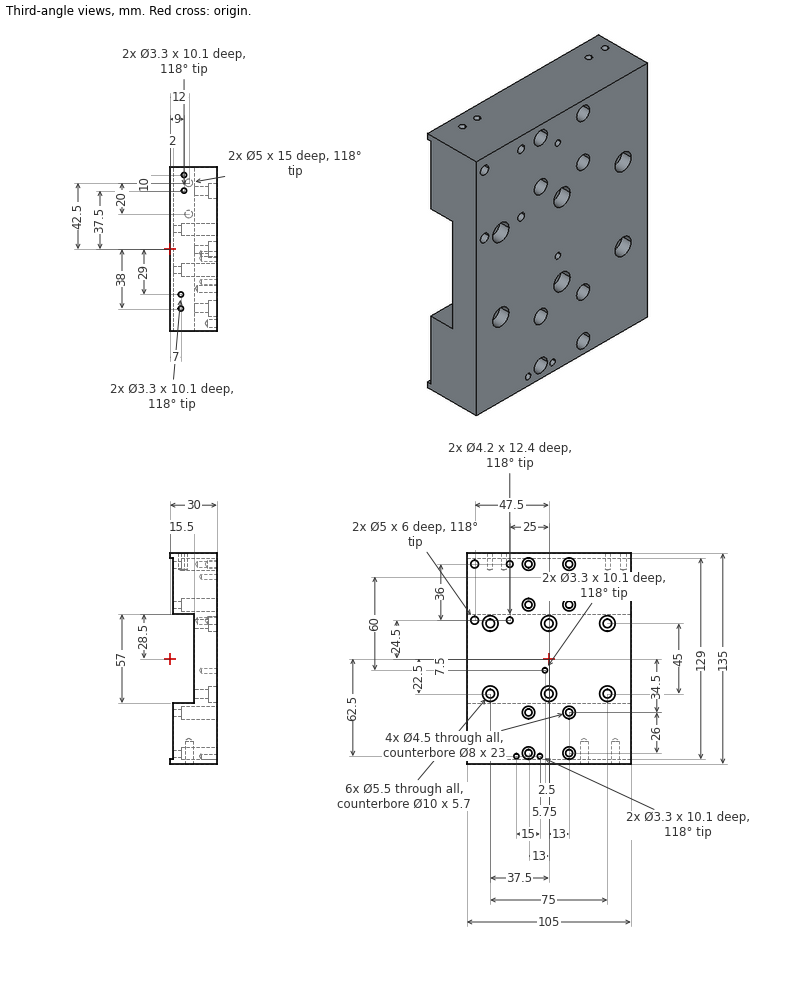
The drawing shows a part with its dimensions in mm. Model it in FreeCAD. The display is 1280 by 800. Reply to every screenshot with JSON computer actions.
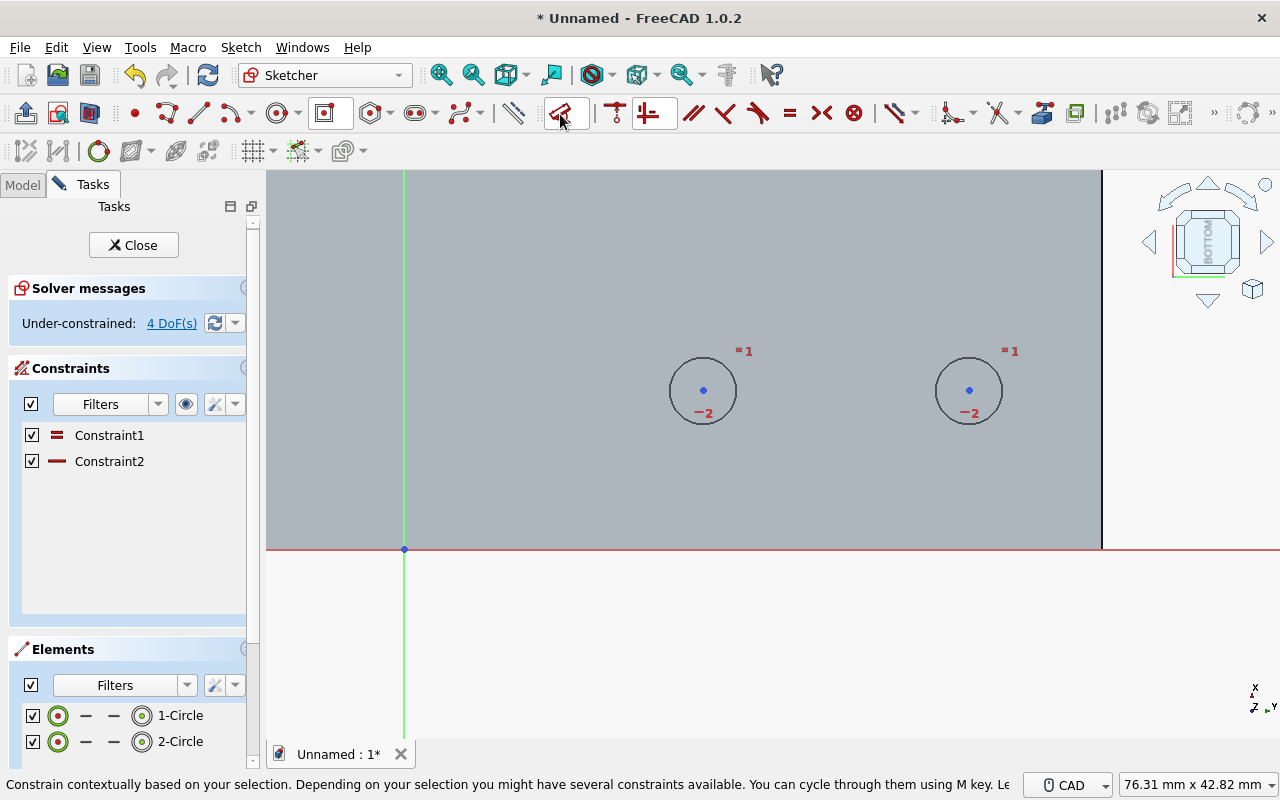
{"action": "left_click", "coordinate": [992, 367]}
{"action": "left_click", "coordinate": [1014, 344]}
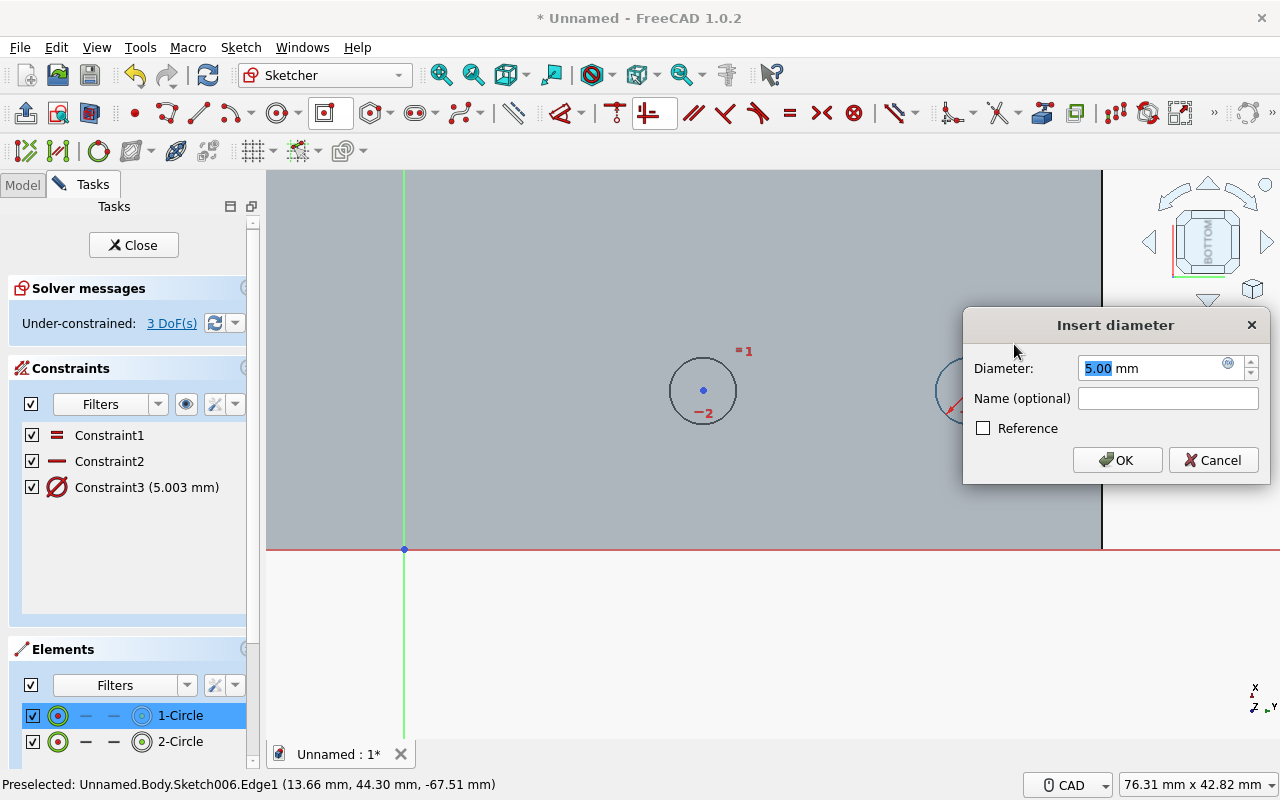
{"action": "type", "text": "5"}
{"action": "key", "text": "Return"}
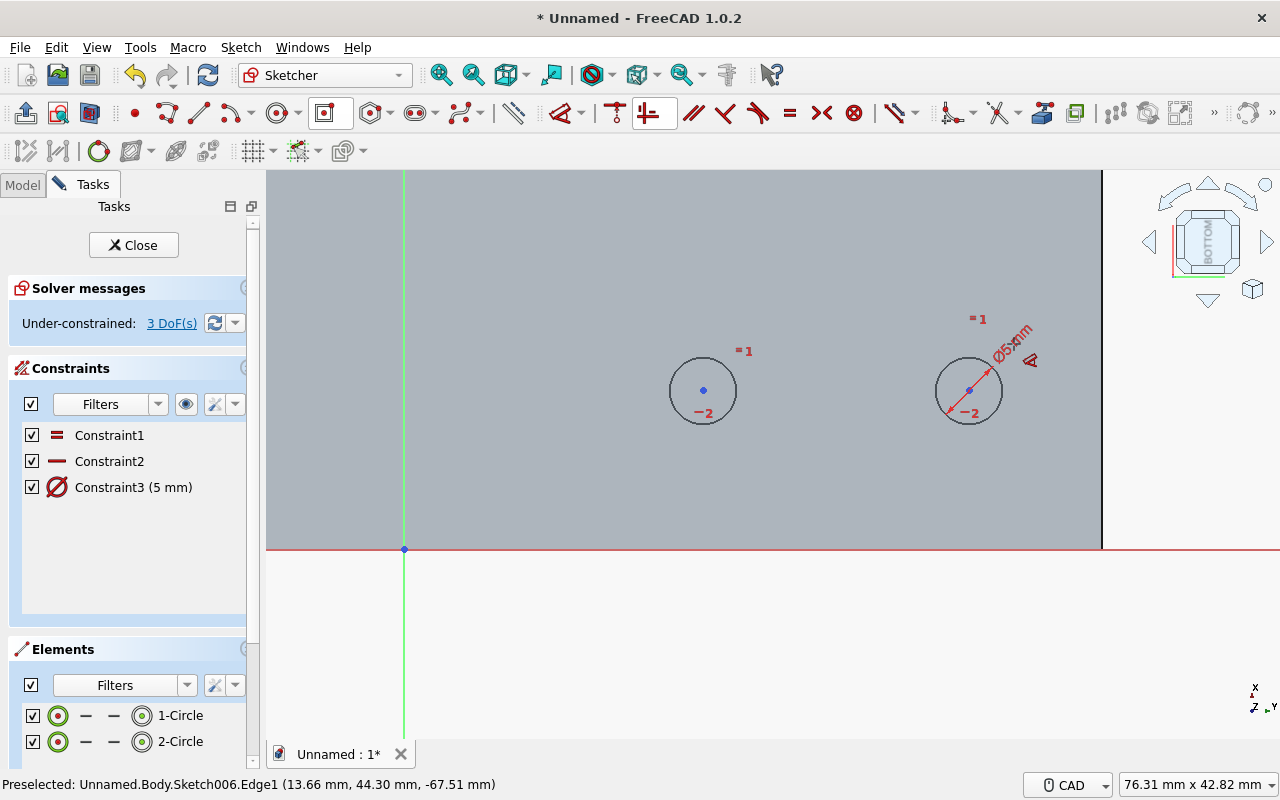
{"action": "left_click", "coordinate": [969, 391]}
{"action": "left_click", "coordinate": [370, 470]}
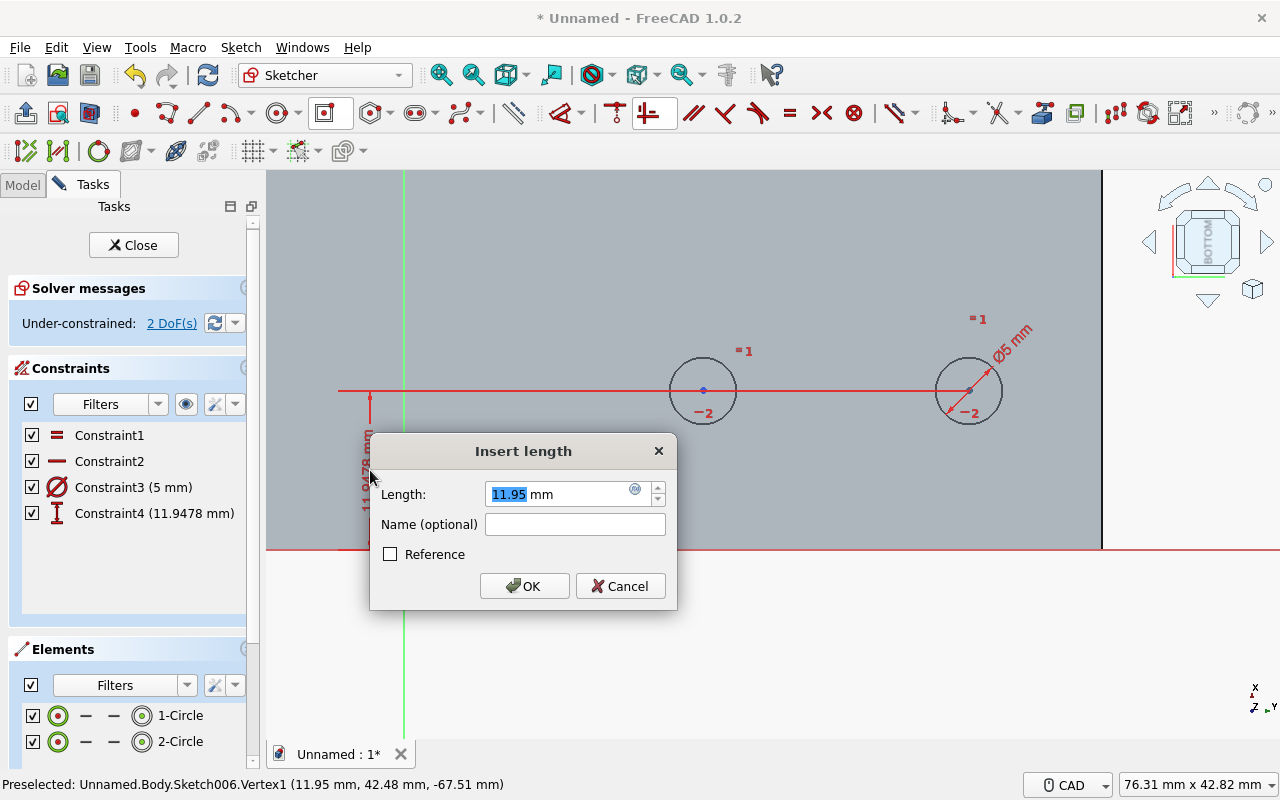
{"action": "type", "text": "12"}
{"action": "key", "text": "Return"}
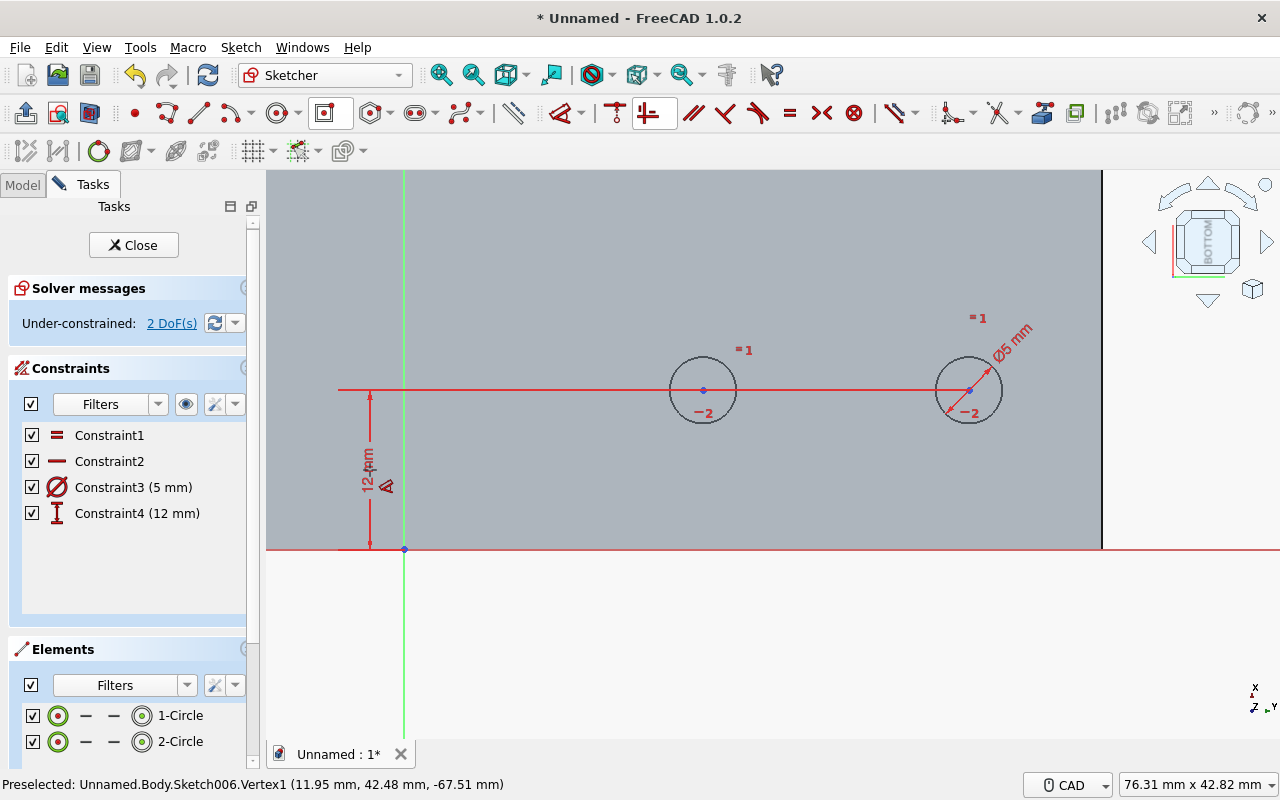
{"action": "left_click", "coordinate": [969, 390]}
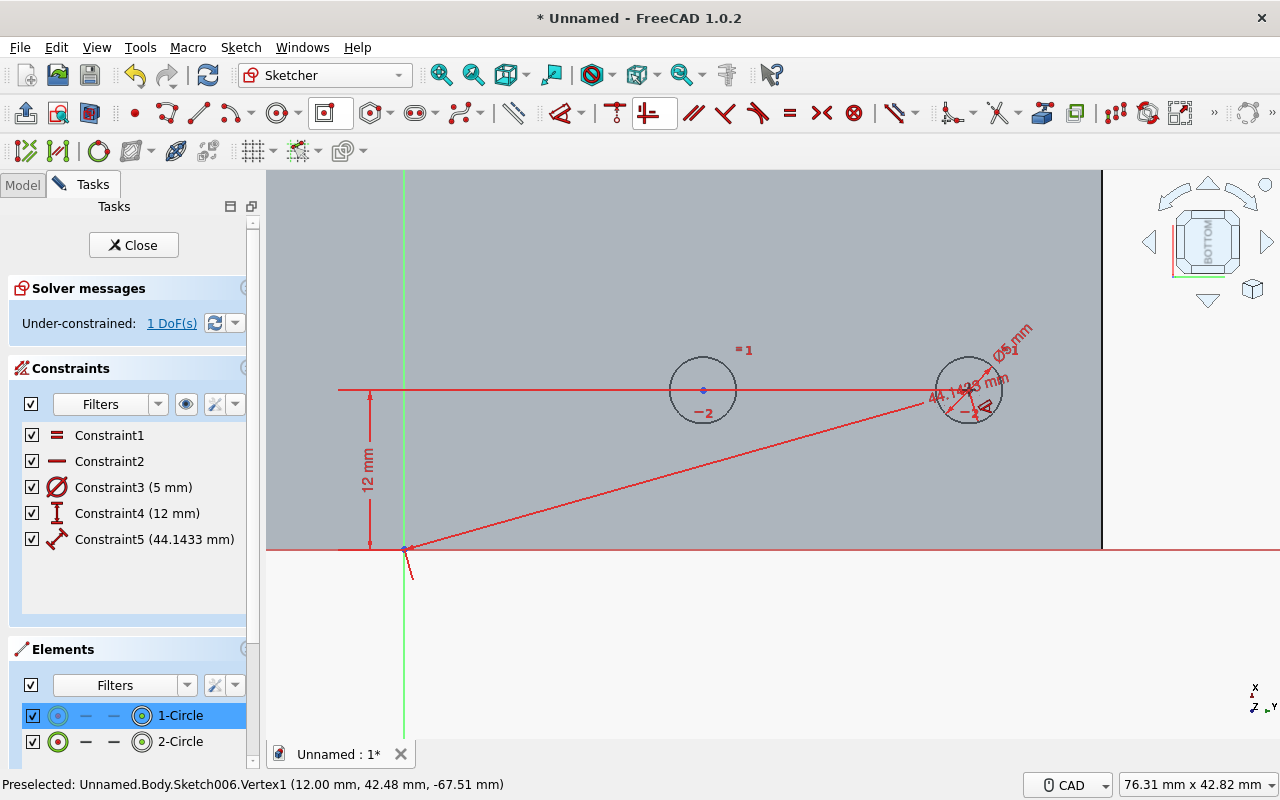
{"action": "left_click", "coordinate": [703, 390]}
{"action": "left_click", "coordinate": [836, 356]}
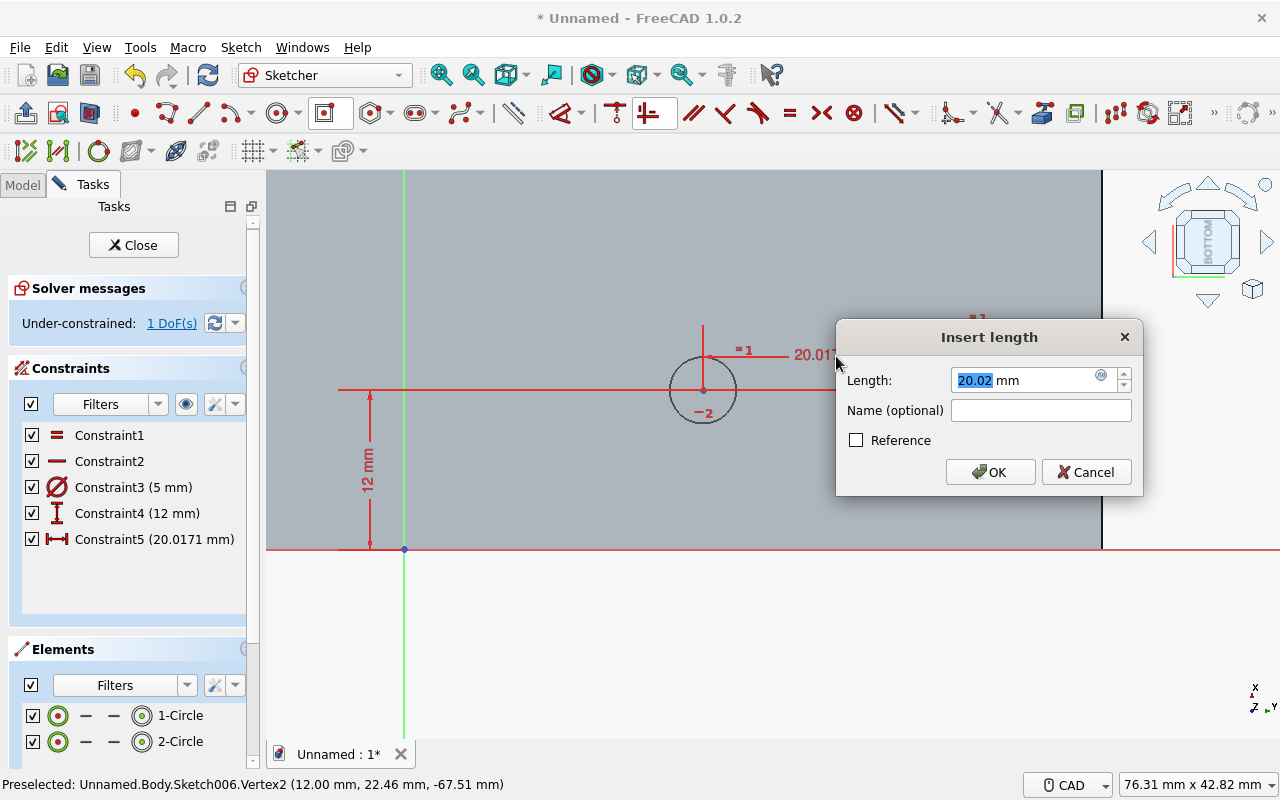
{"action": "type", "text": "20"}
{"action": "key", "text": "Return"}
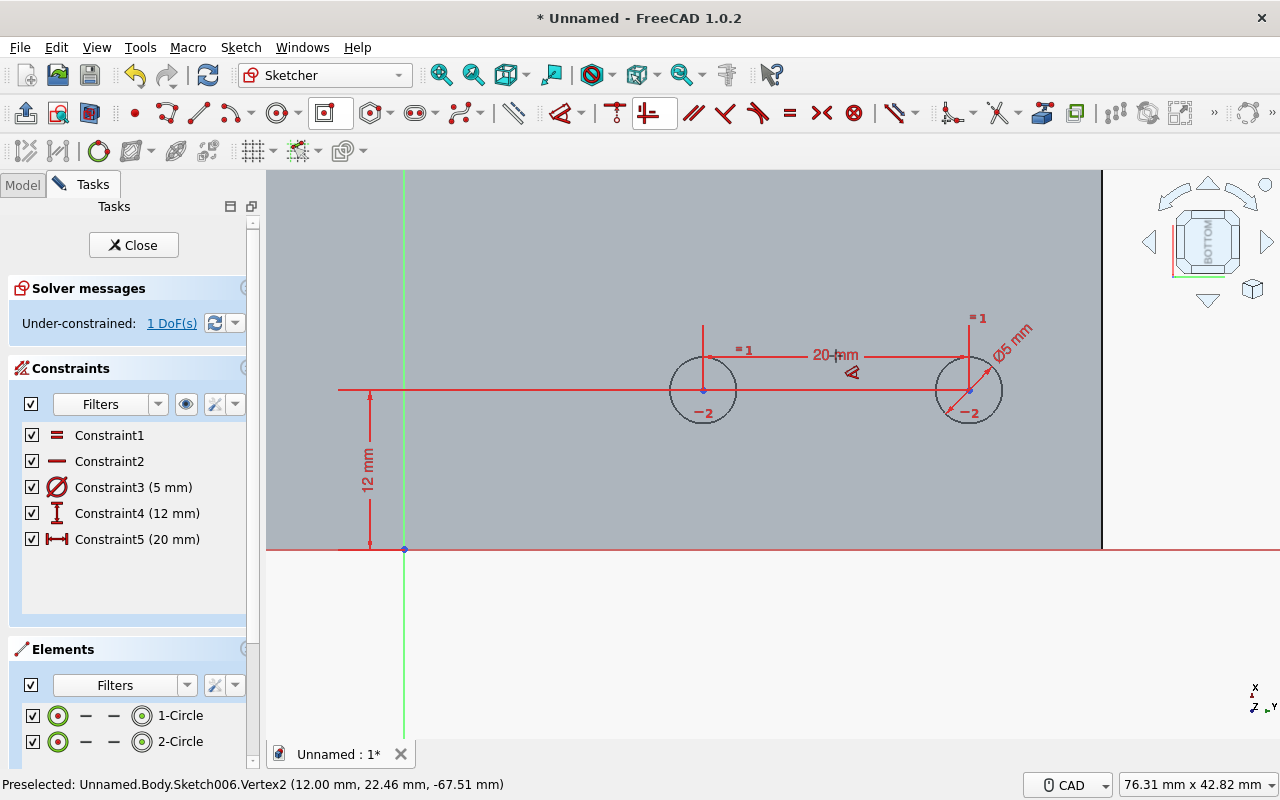
{"action": "left_click", "coordinate": [969, 390]}
{"action": "left_click", "coordinate": [687, 584]}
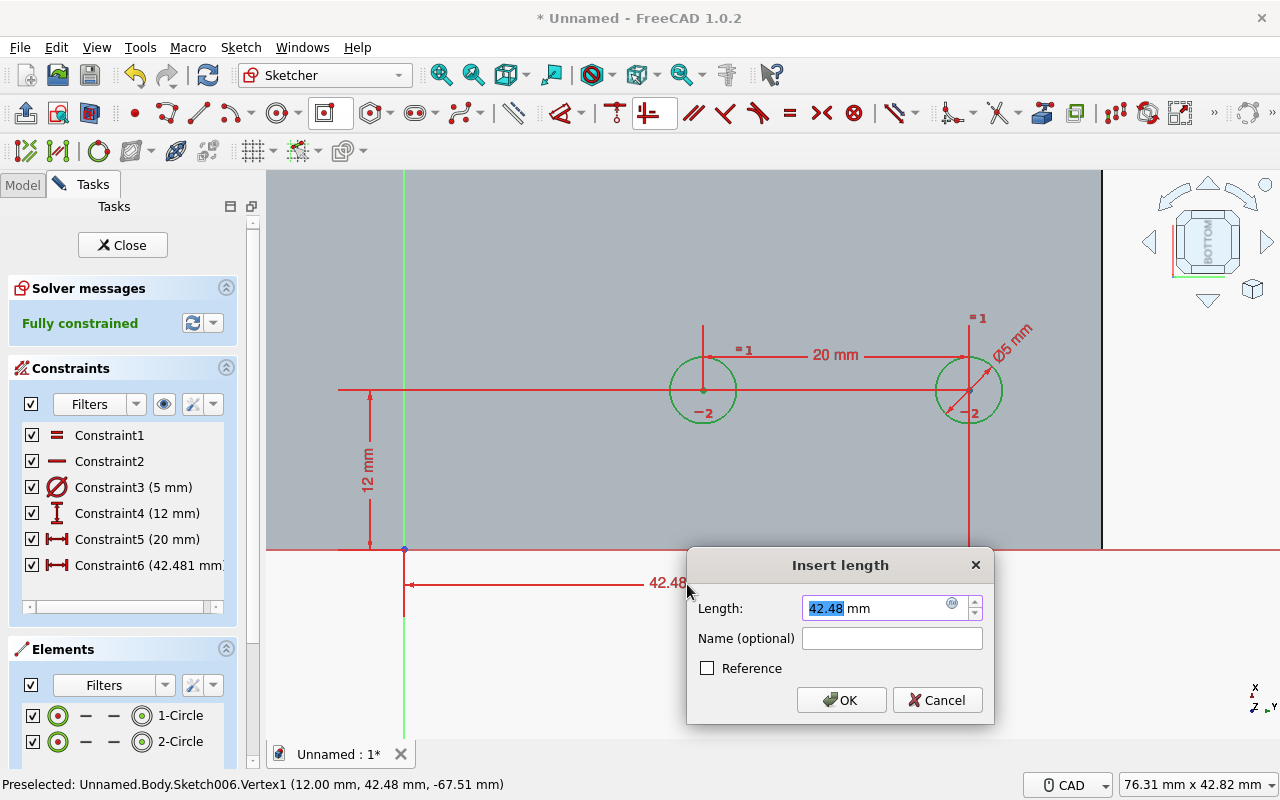
{"action": "type", "text": "42.5"}
{"action": "key", "text": "Return"}
{"action": "key", "text": "Escape"}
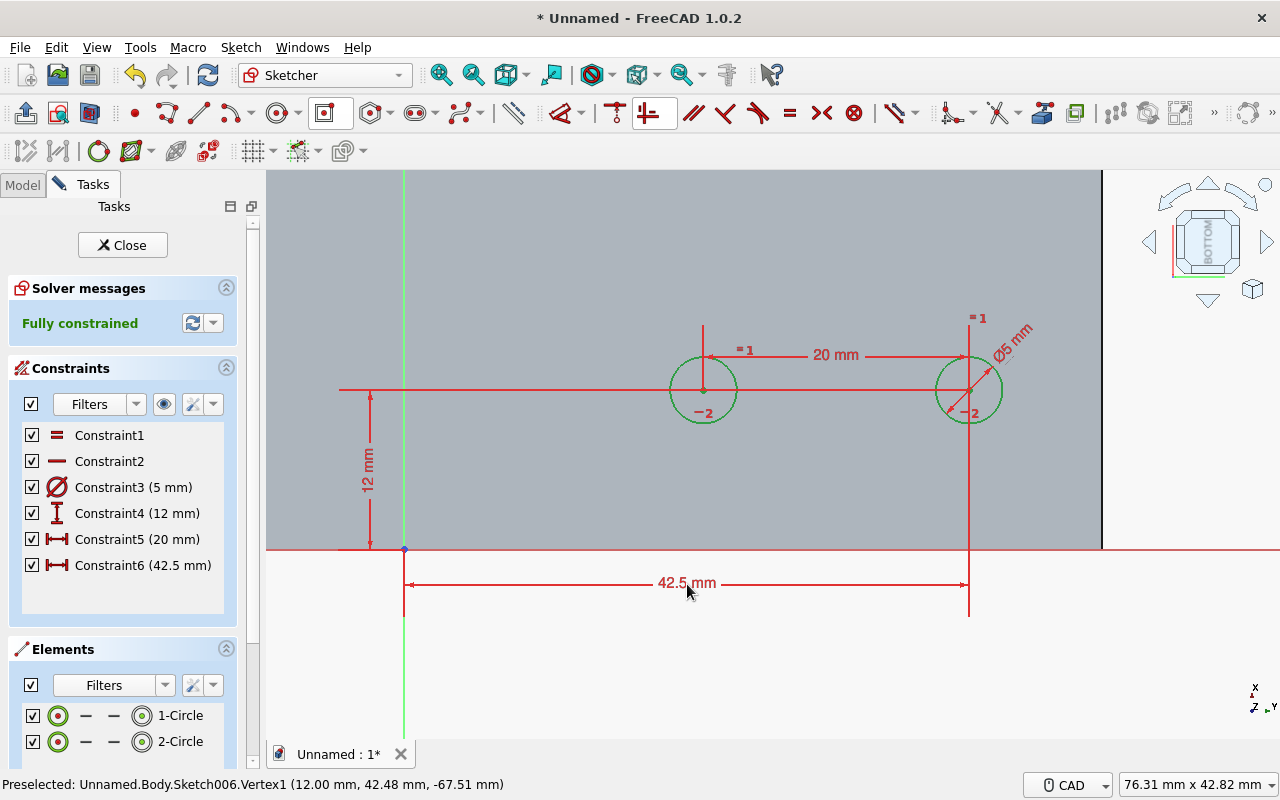
{"action": "left_click", "coordinate": [123, 245]}